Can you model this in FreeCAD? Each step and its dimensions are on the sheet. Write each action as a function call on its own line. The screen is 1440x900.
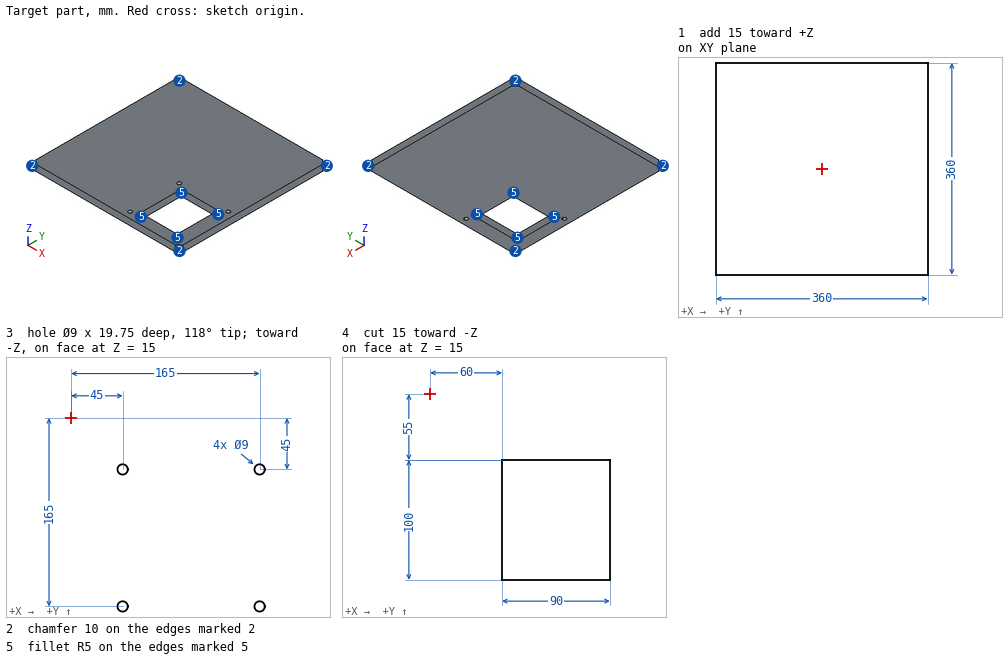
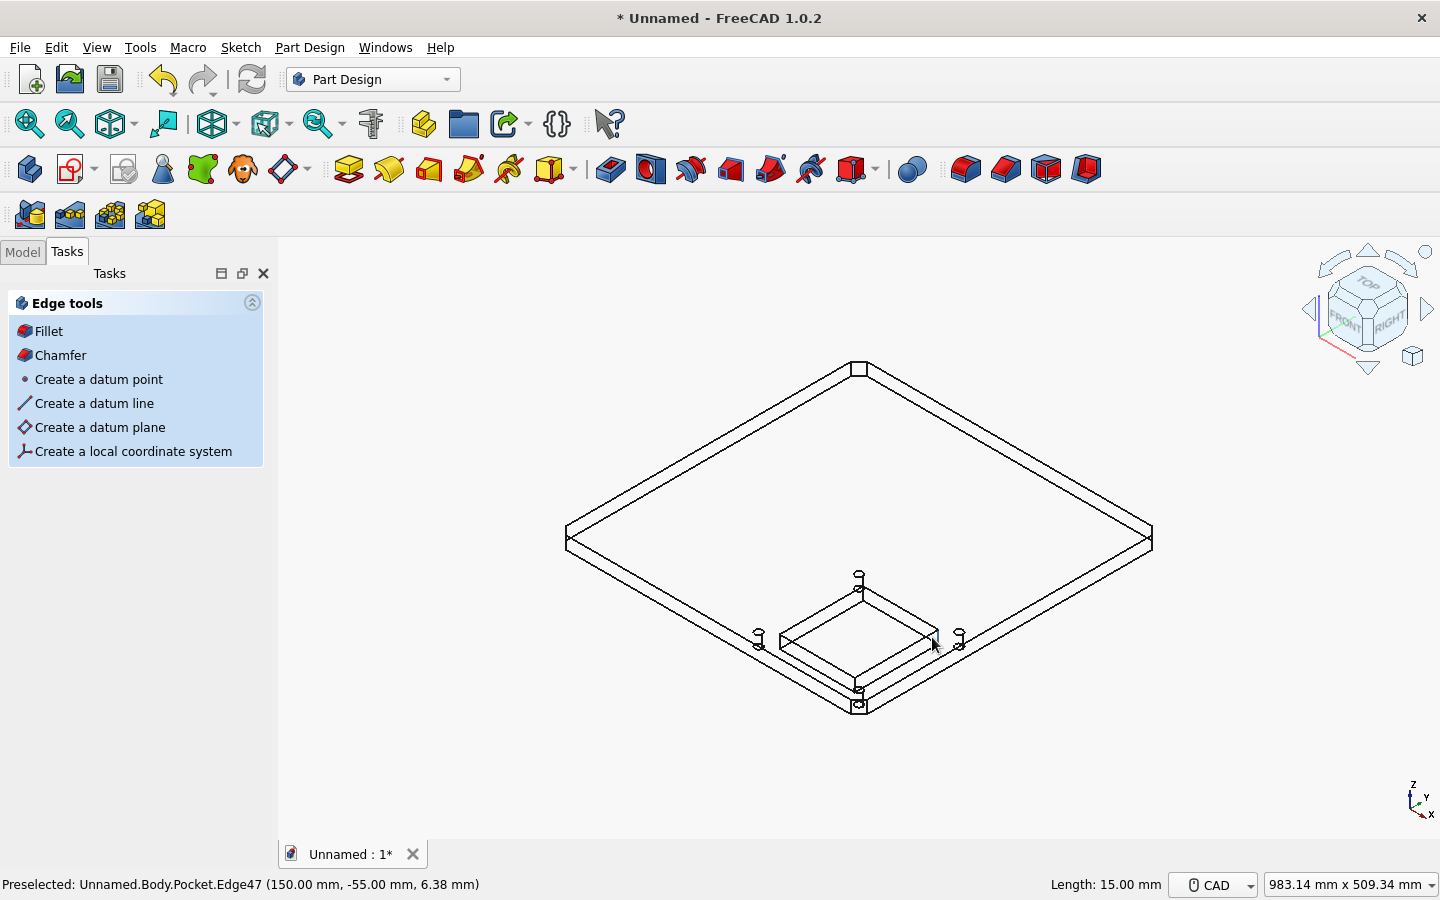
click(780, 642, ctrl)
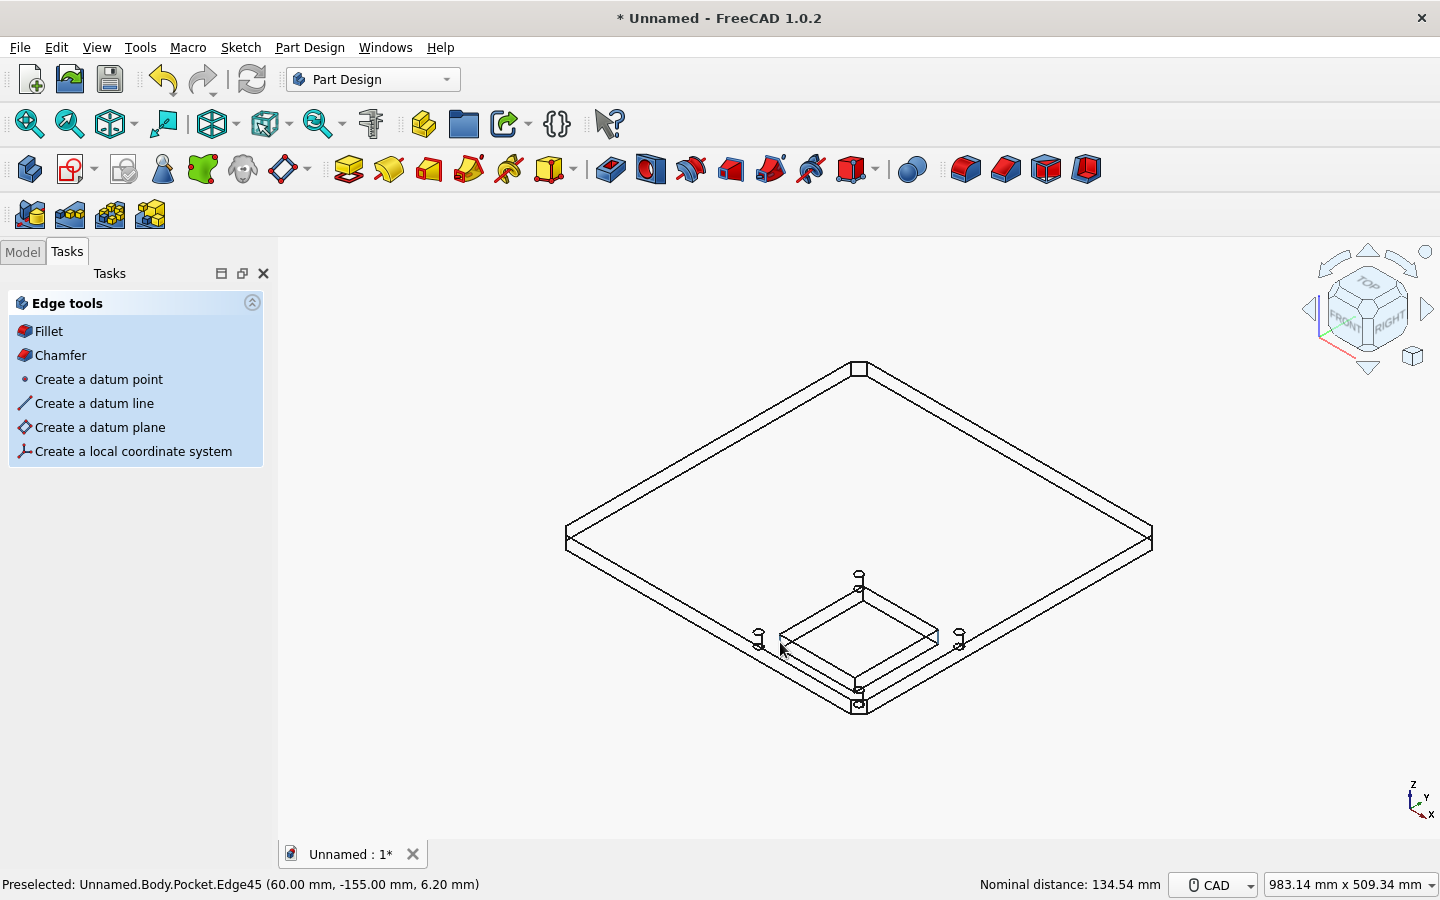
click(863, 594, ctrl)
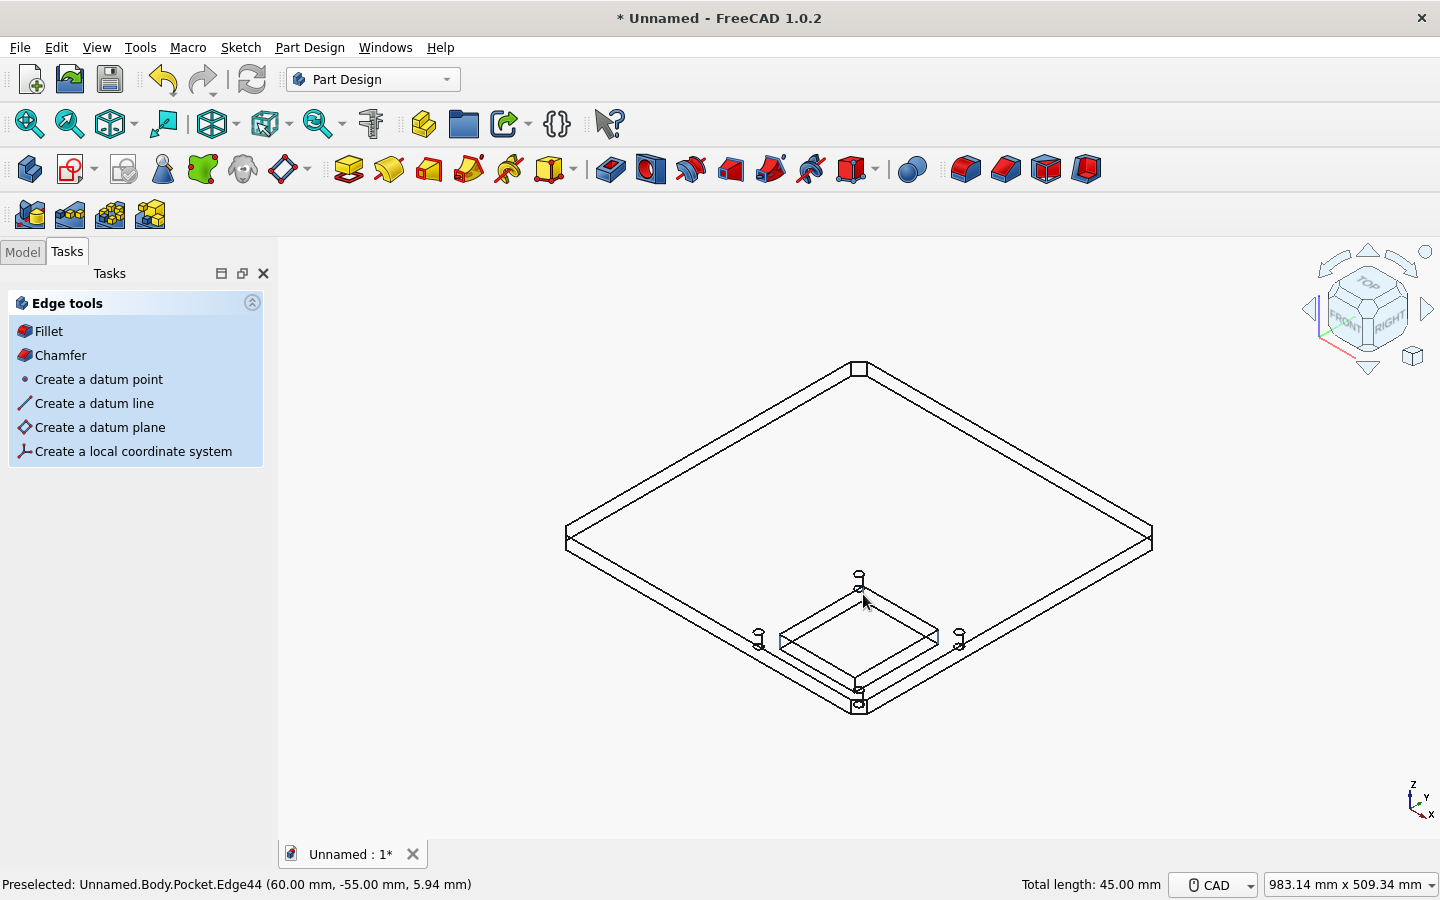
scroll(855, 684, up, 5)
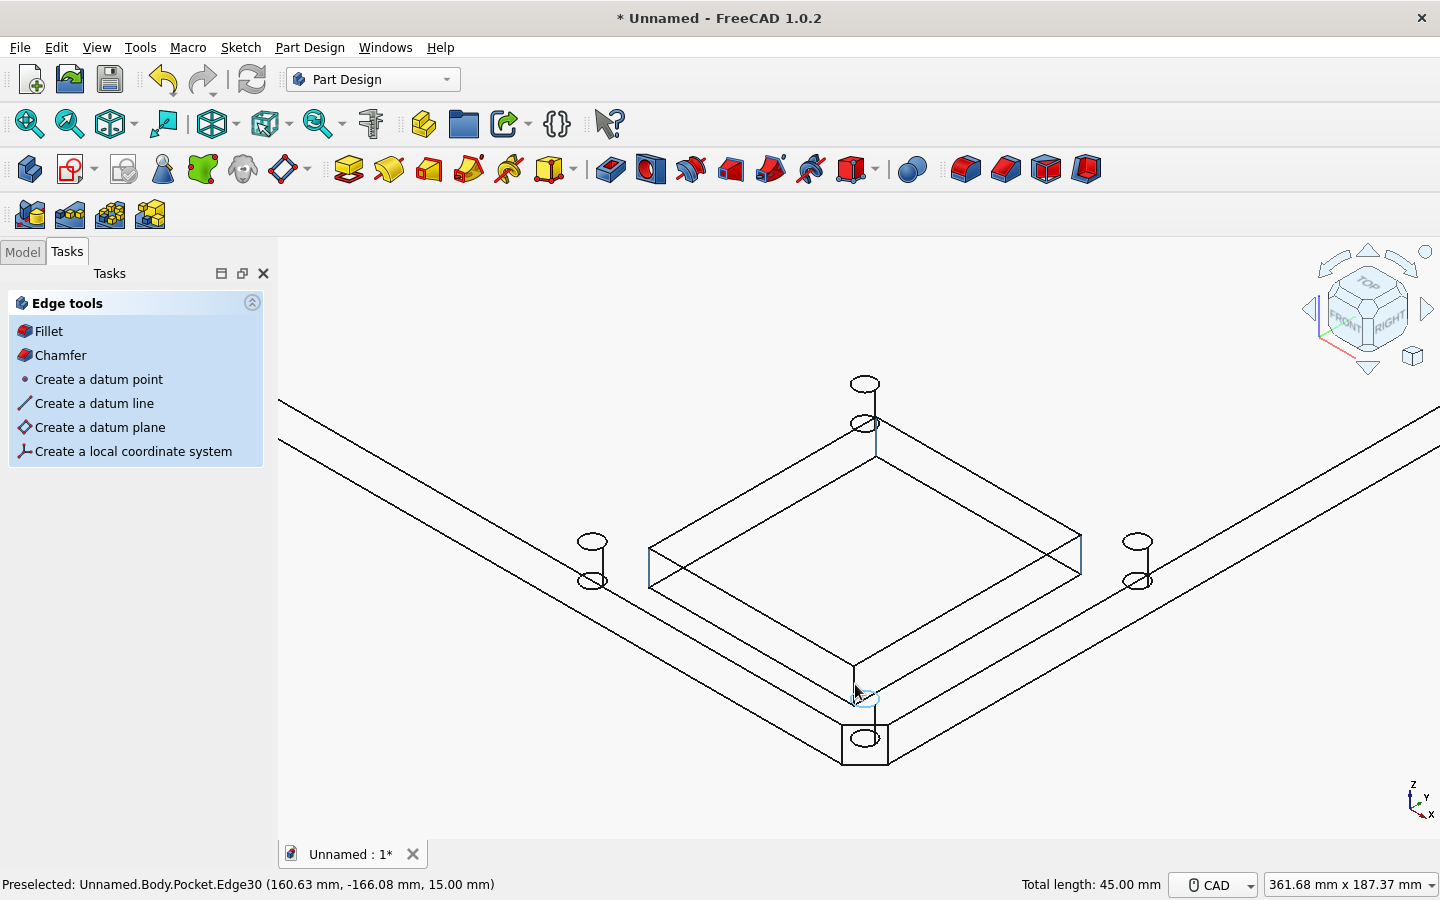
click(854, 685, ctrl)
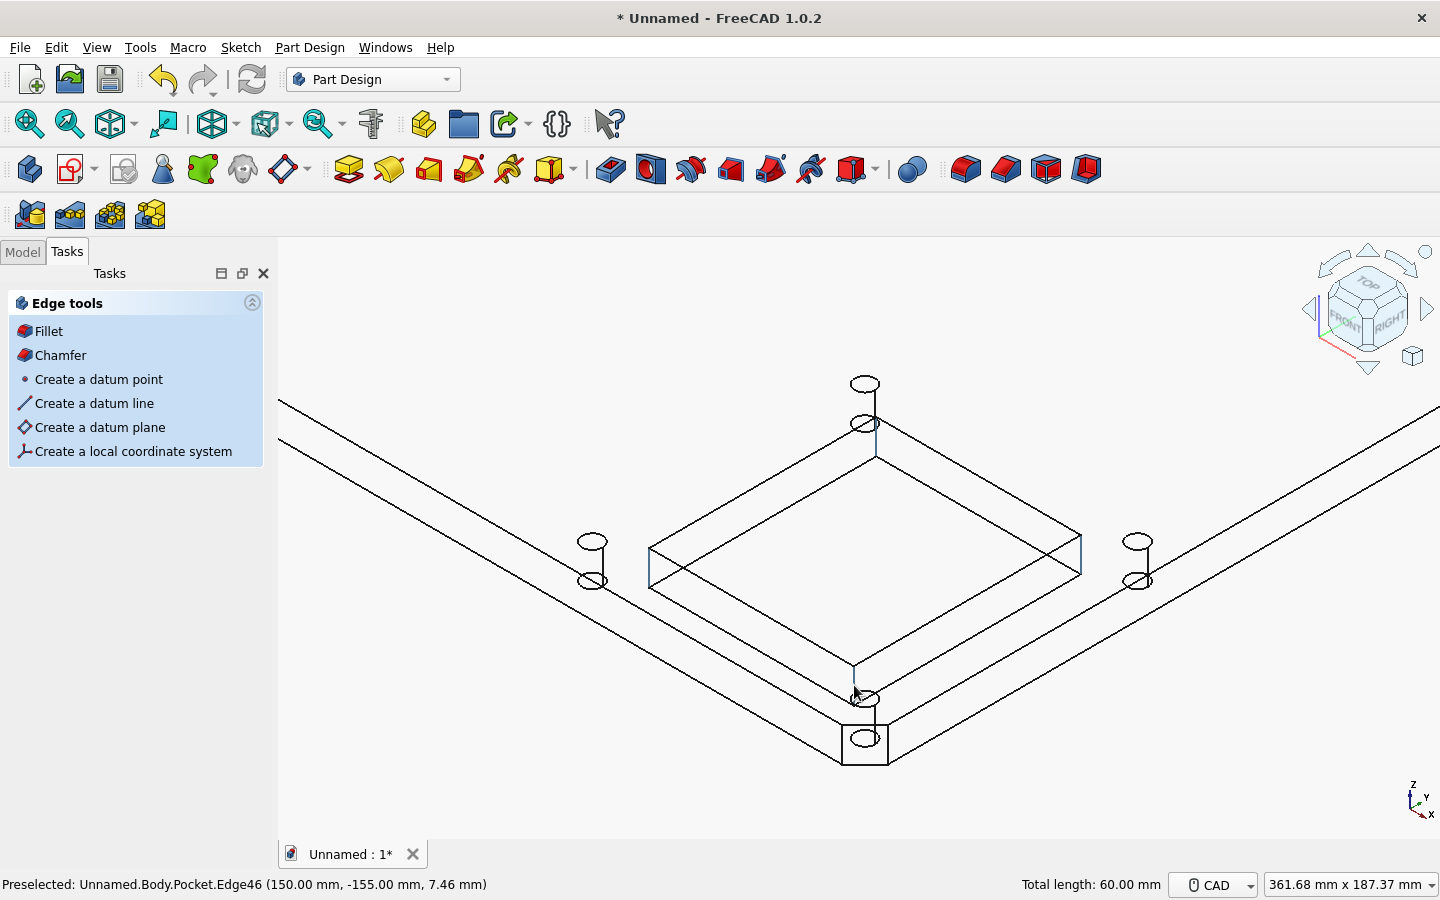
key(v)
key(1)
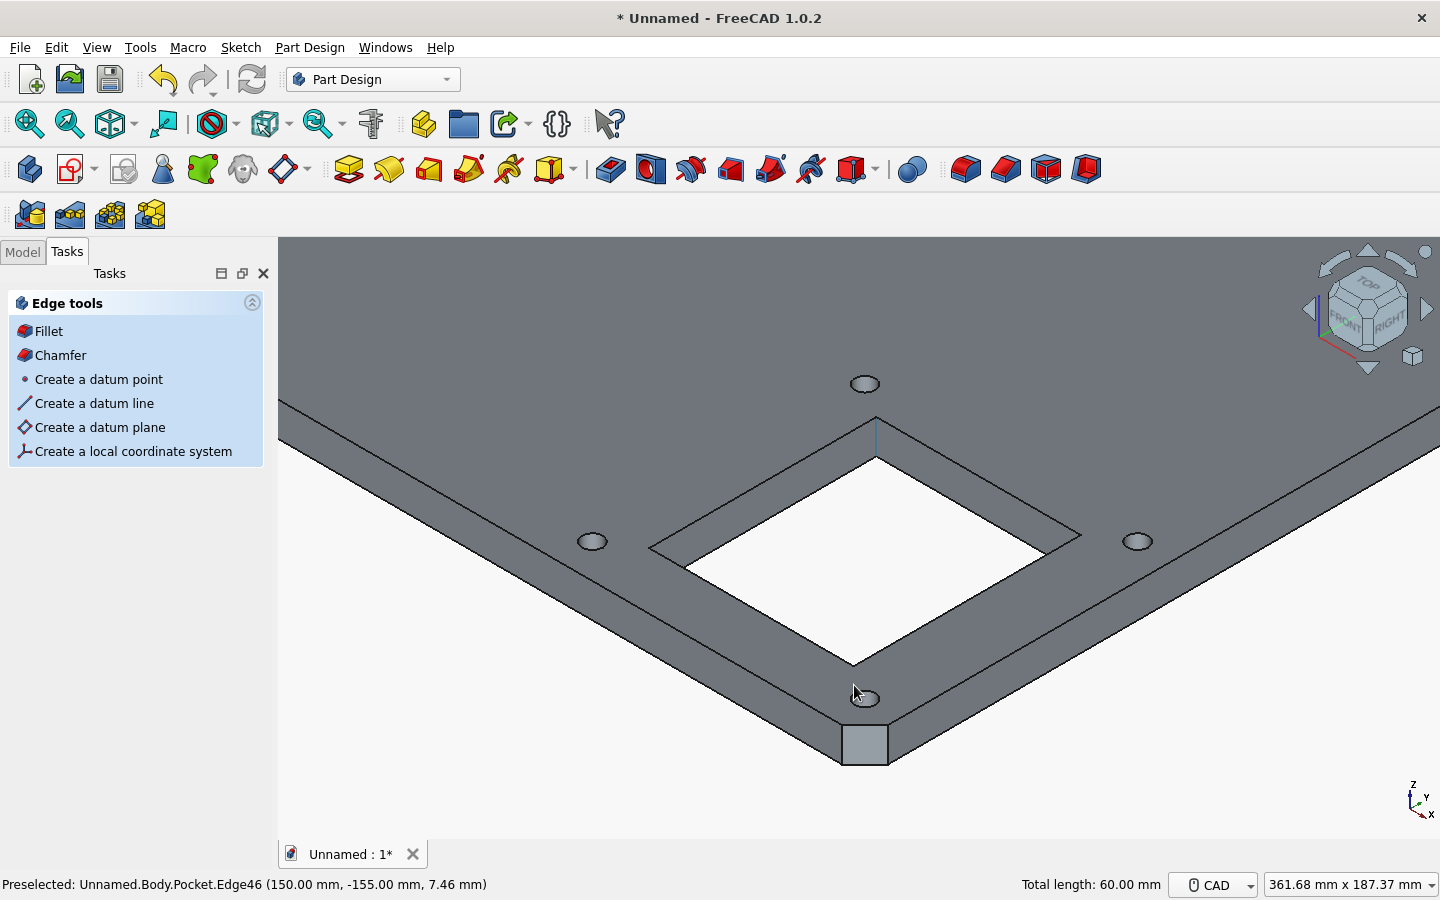
click(966, 170)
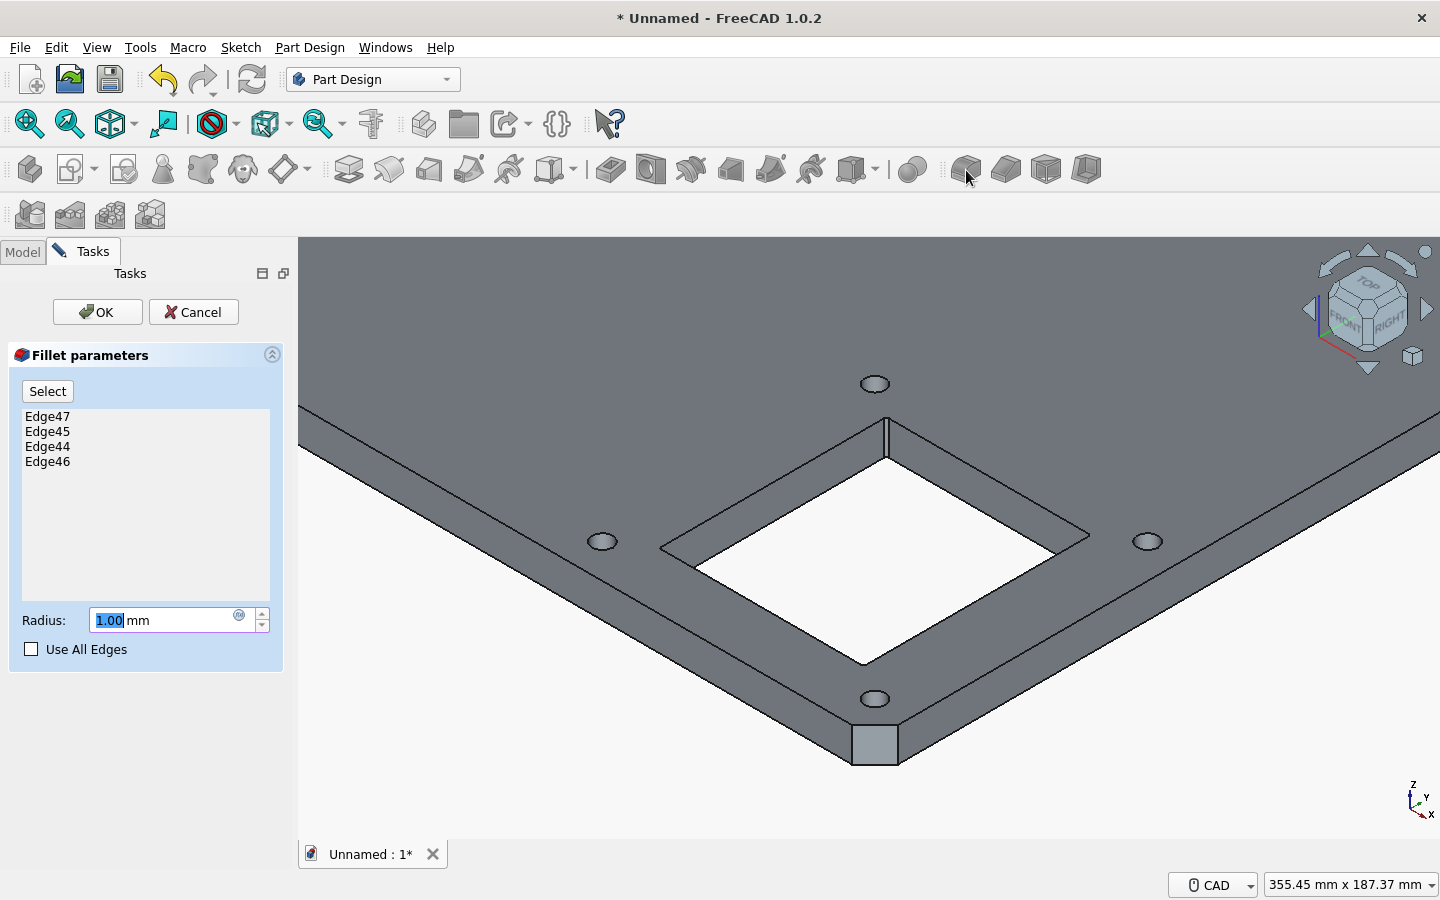
text(5)
key(Tab)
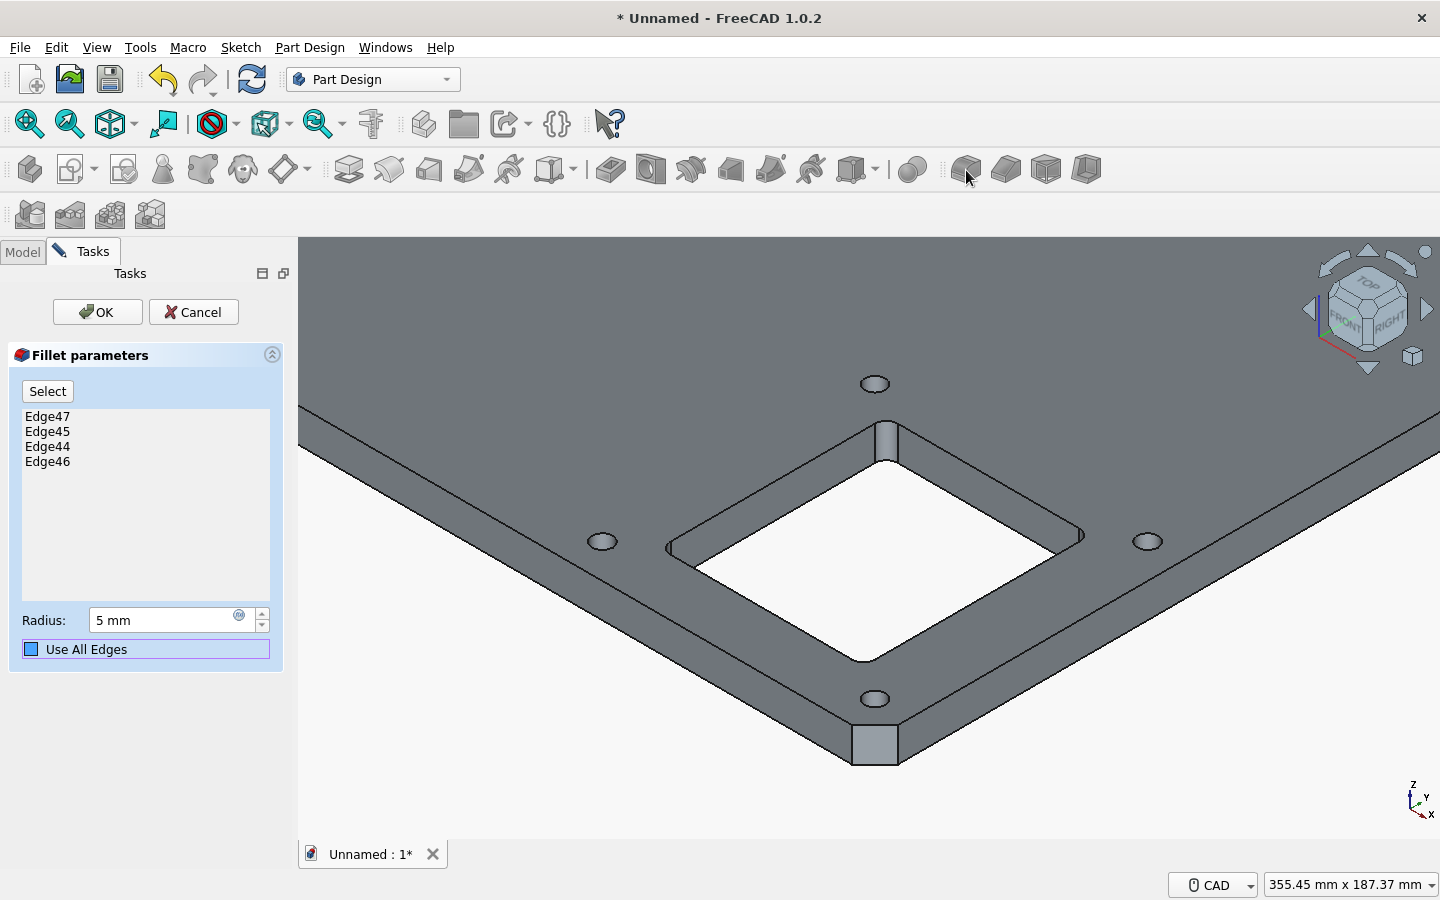
click(98, 312)